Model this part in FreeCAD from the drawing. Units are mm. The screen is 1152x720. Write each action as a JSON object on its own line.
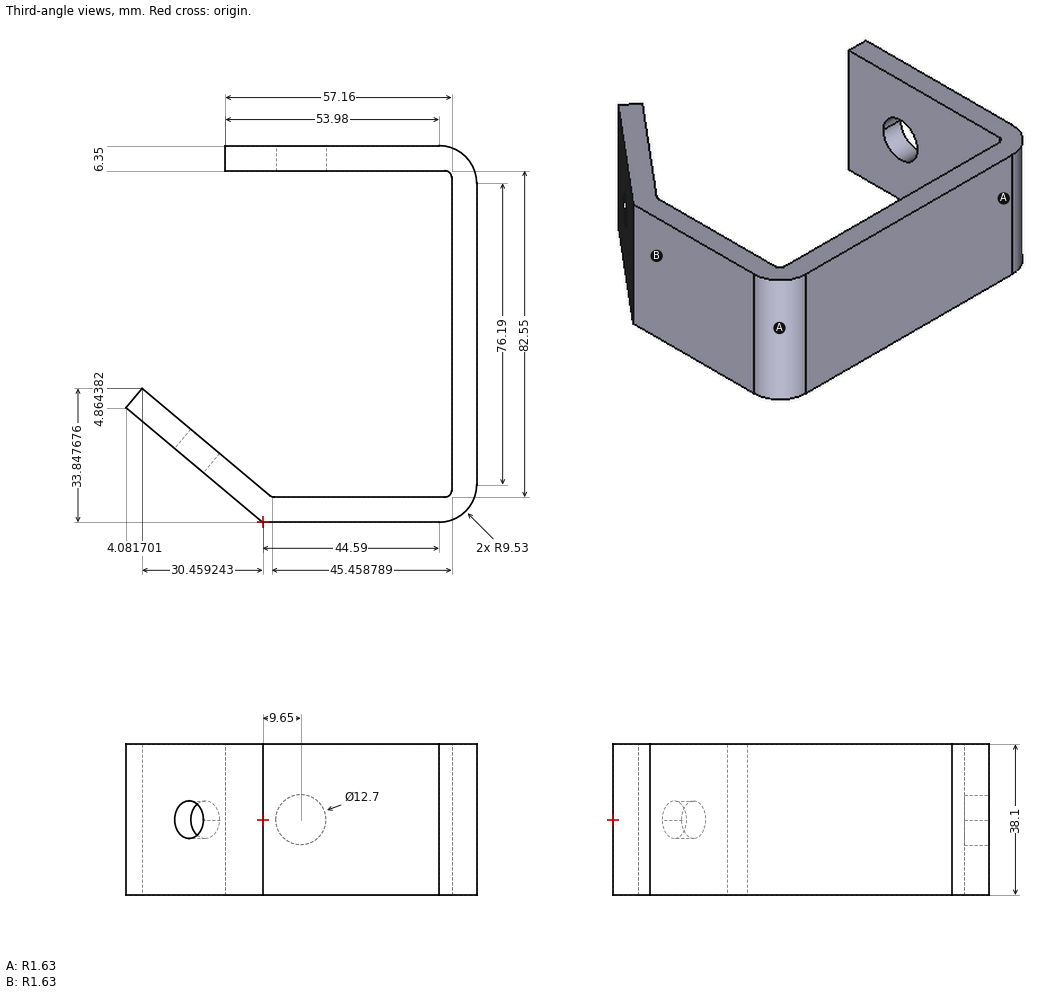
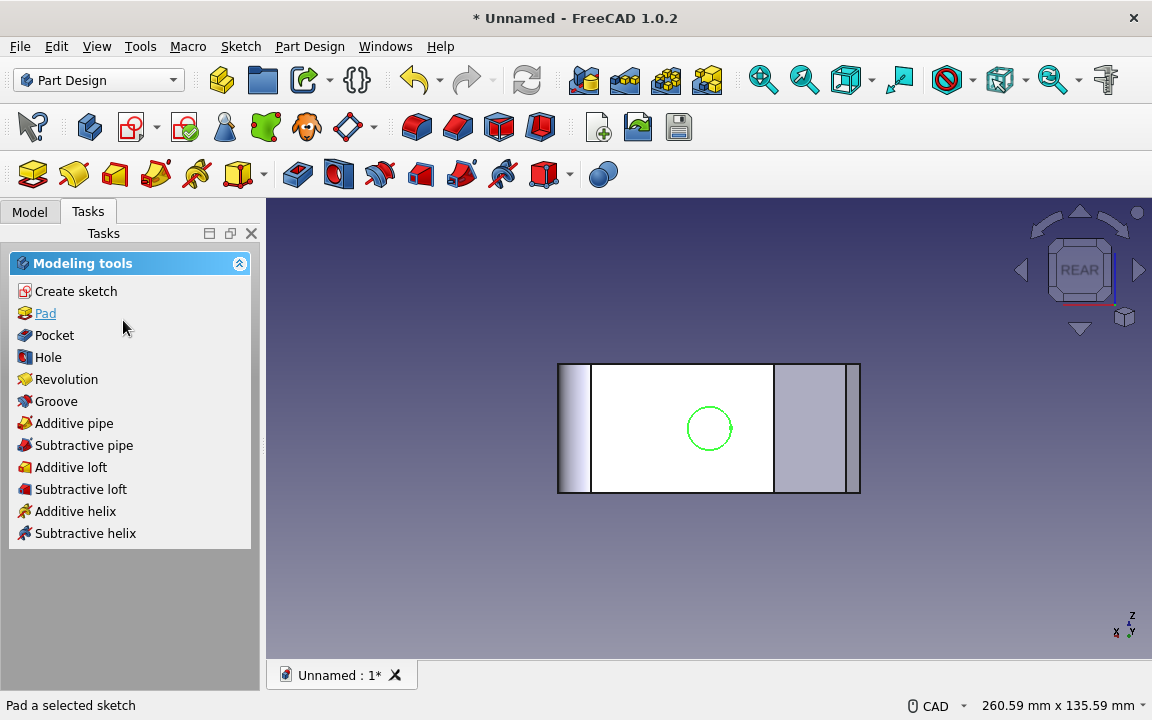
{"action": "left_click", "coordinate": [298, 174]}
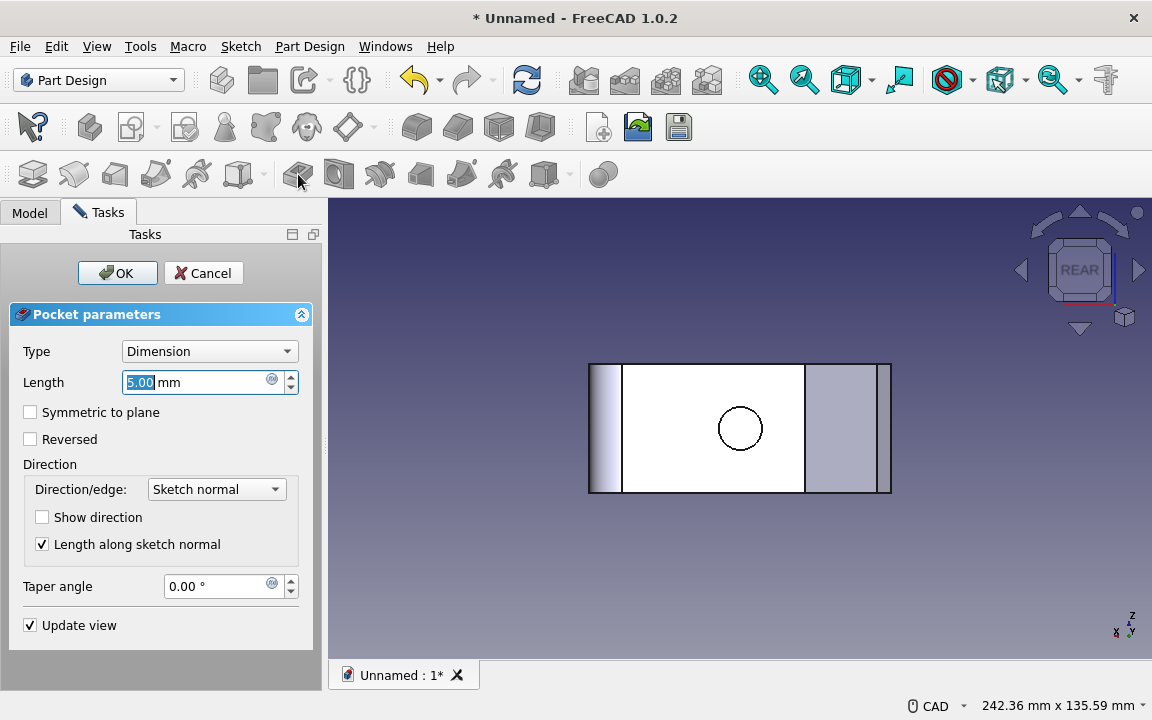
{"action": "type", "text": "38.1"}
{"action": "key", "text": "Tab"}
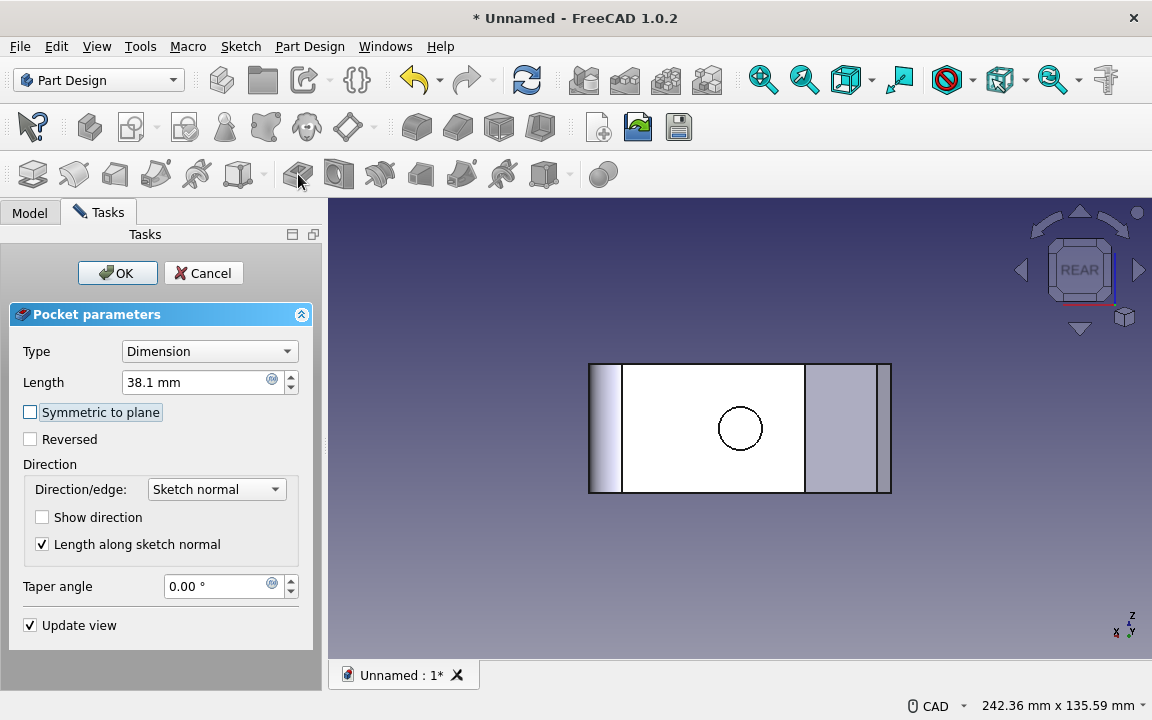
{"action": "left_click", "coordinate": [31, 412]}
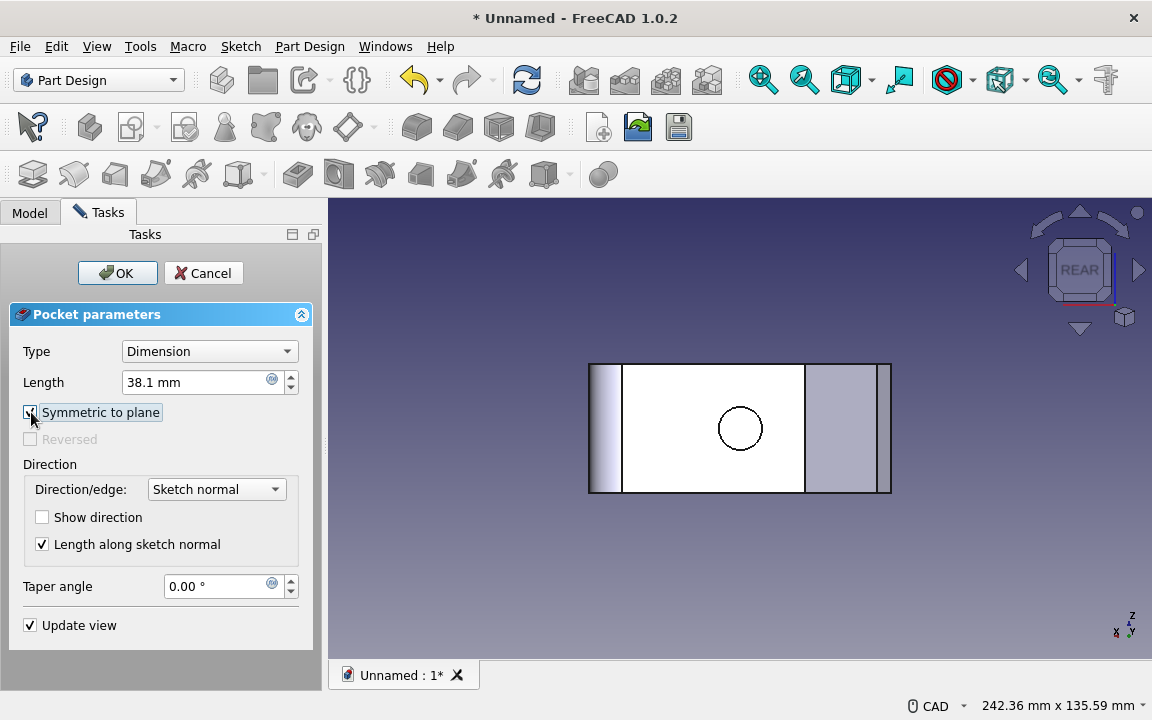
{"action": "left_click", "coordinate": [118, 273]}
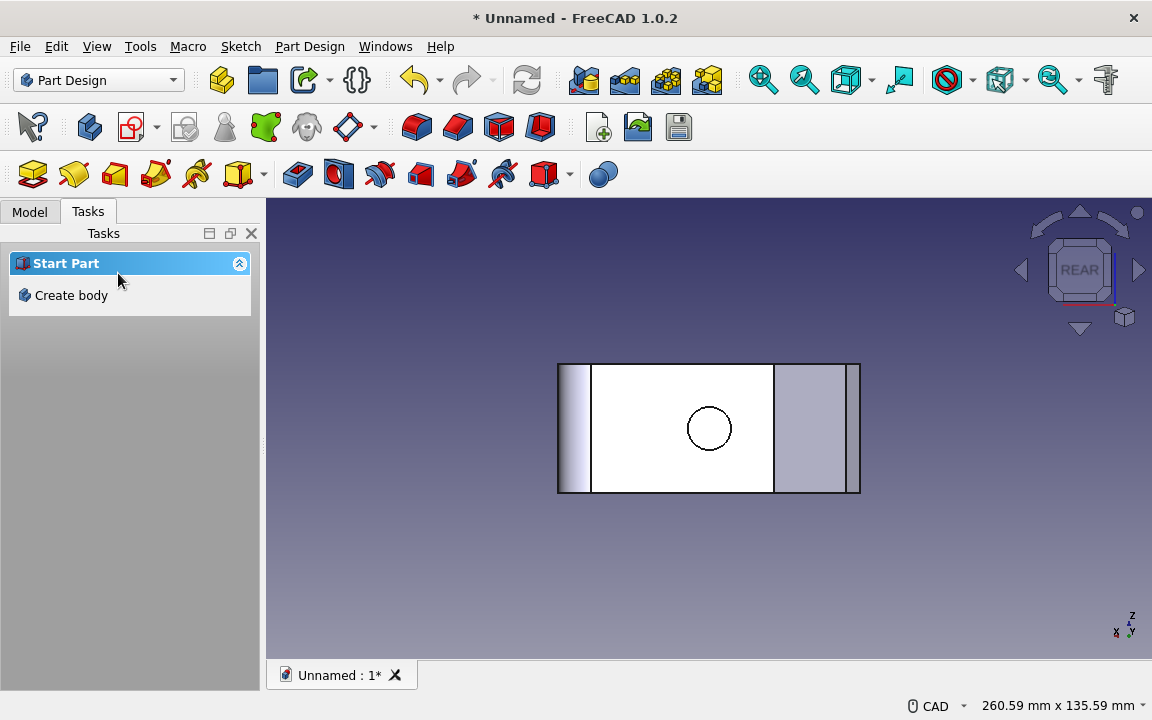
{"action": "left_click", "coordinate": [764, 80]}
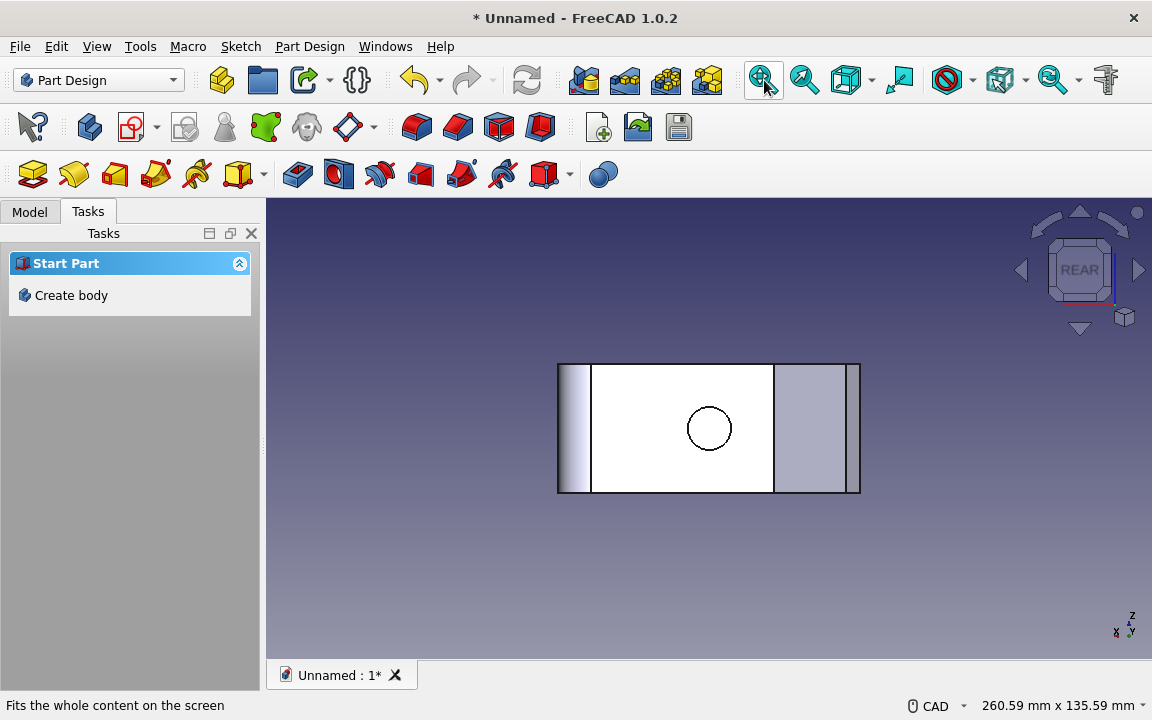
{"action": "key", "text": "1"}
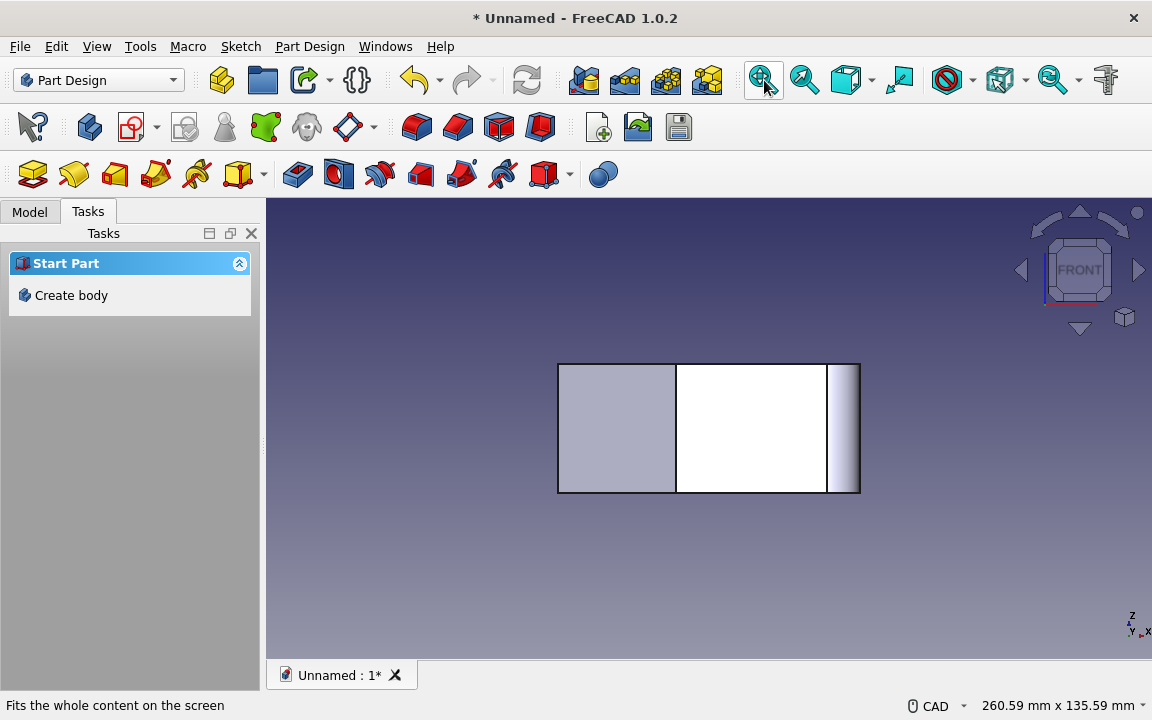
{"action": "key", "text": "v f"}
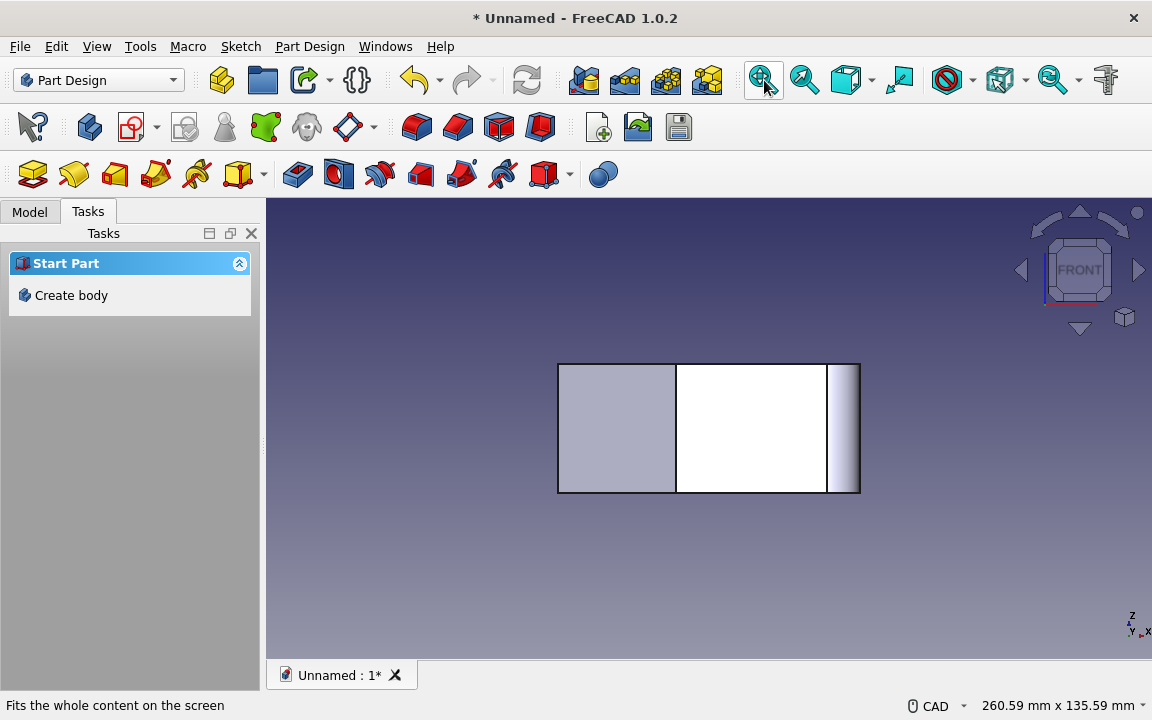
{"action": "left_click", "coordinate": [617, 428]}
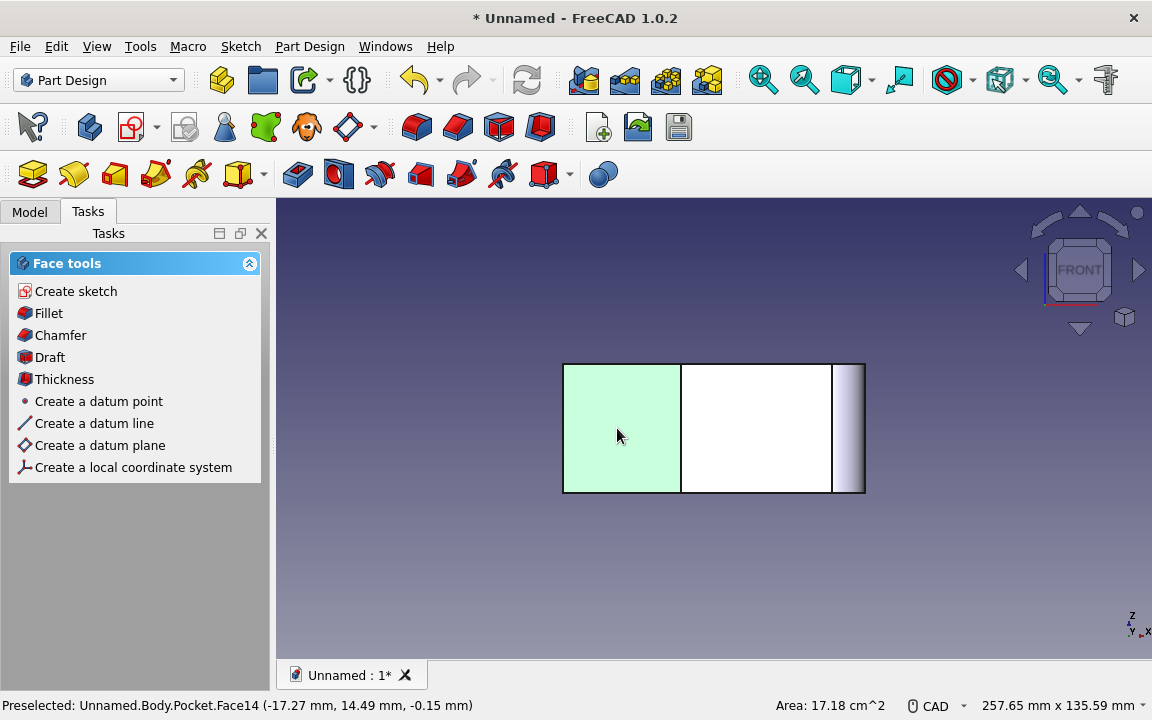
{"action": "left_click", "coordinate": [130, 128]}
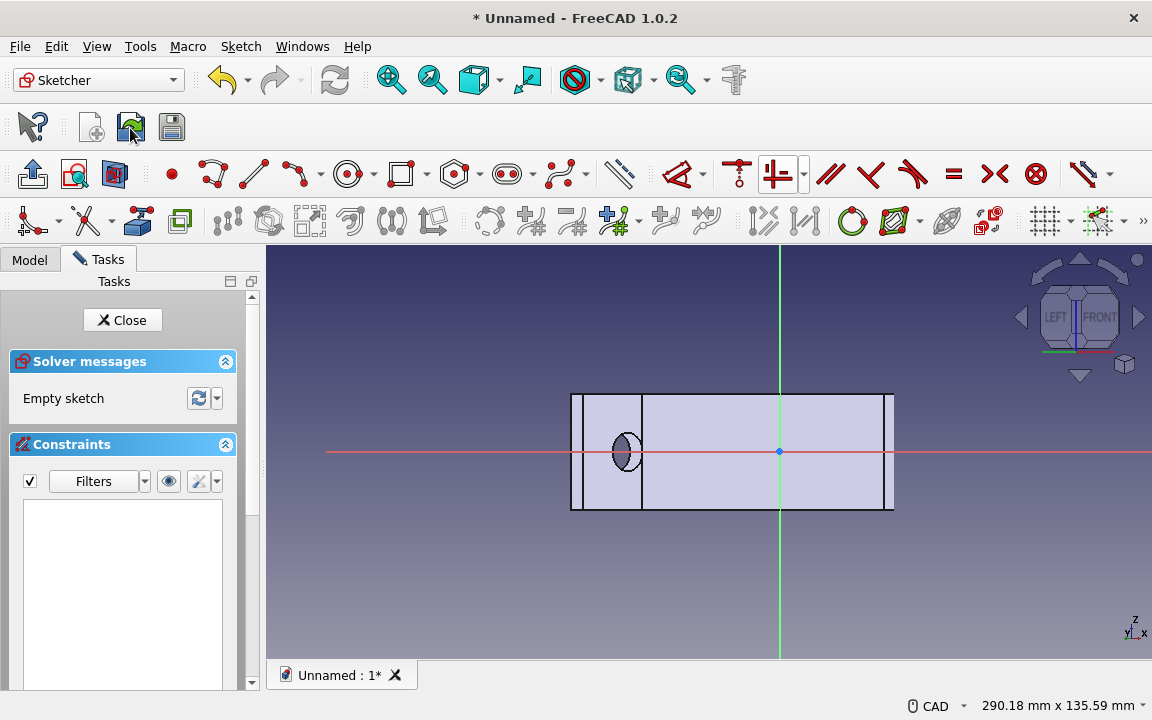
{"action": "key", "text": "q s"}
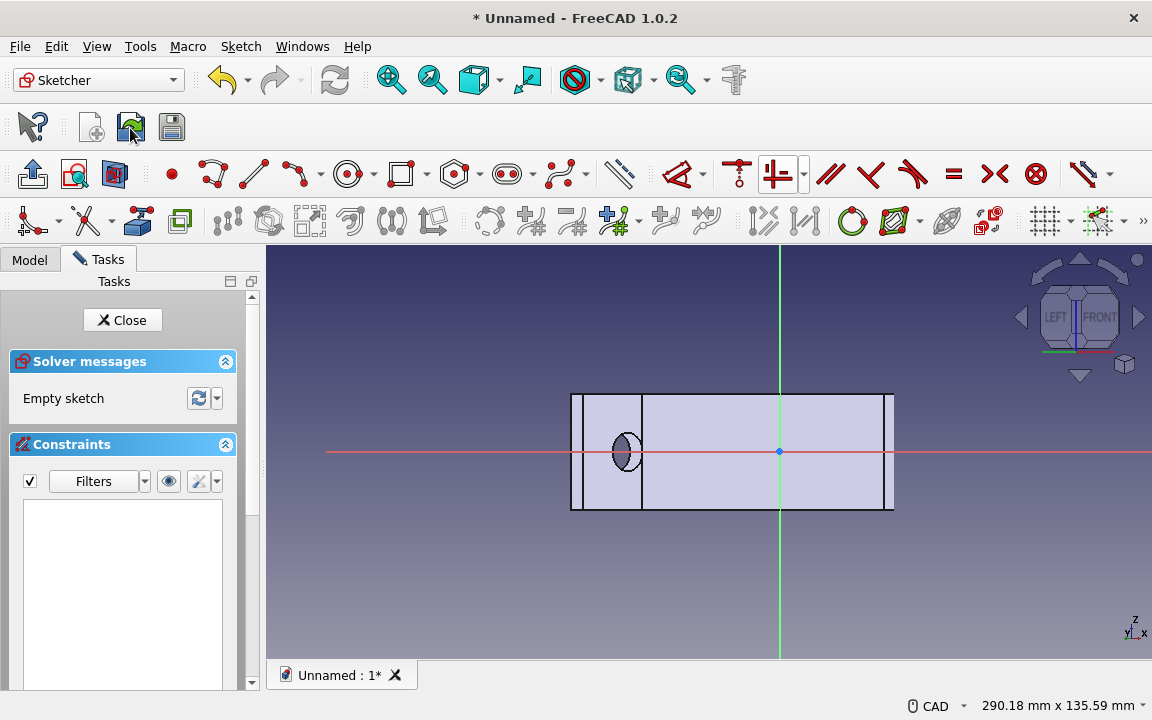
{"action": "scroll", "coordinate": [714, 452], "scroll_direction": "up", "scroll_amount": 11}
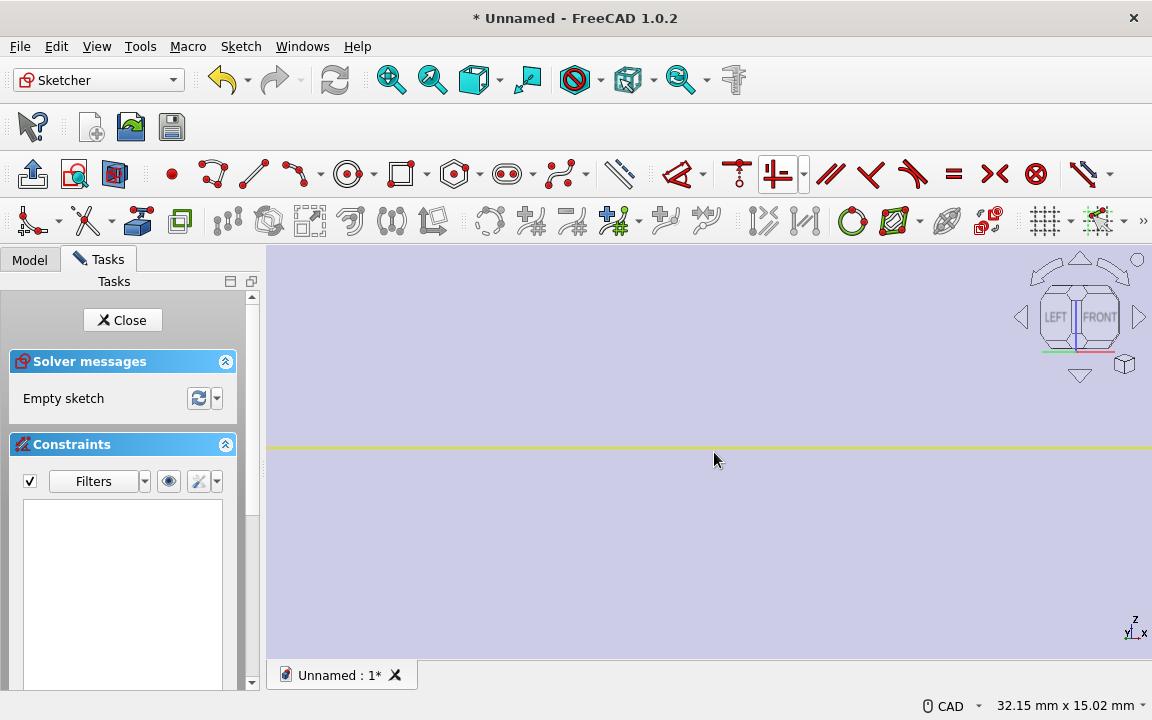
{"action": "key", "text": "g c"}